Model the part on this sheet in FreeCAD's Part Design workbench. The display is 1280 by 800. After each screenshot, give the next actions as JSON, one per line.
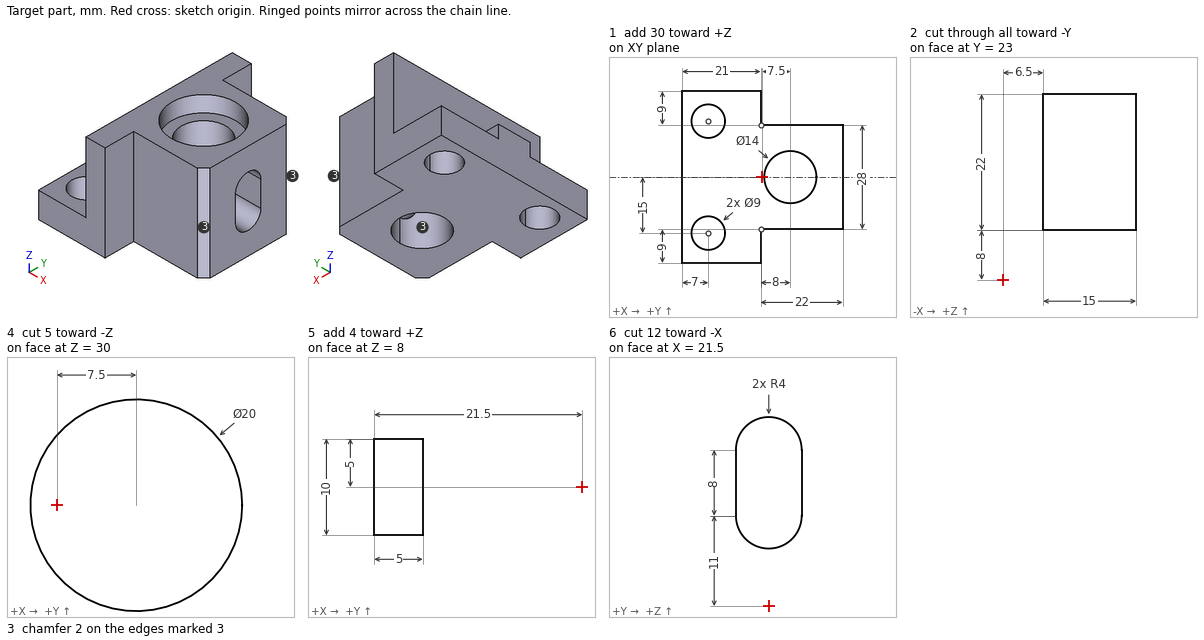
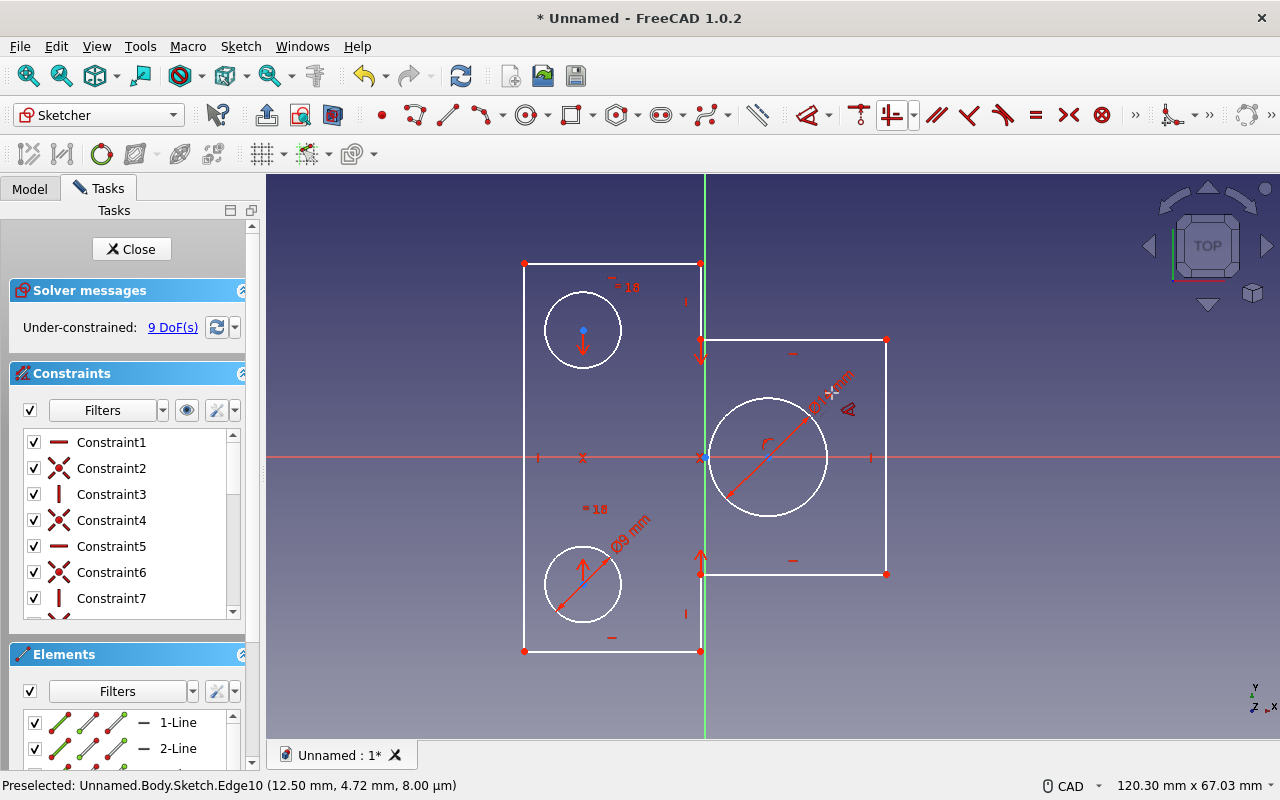
{"action": "scroll", "coordinate": [701, 317], "scroll_direction": "up", "scroll_amount": 6}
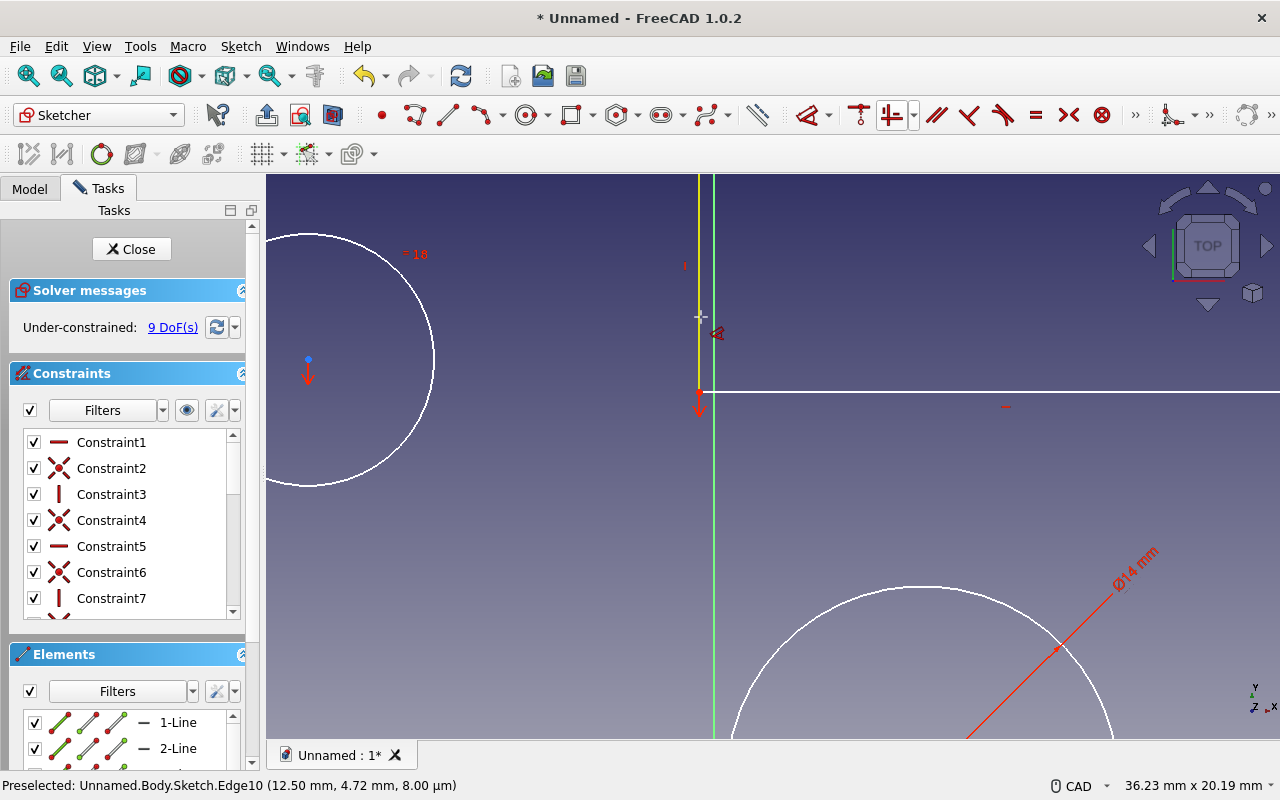
{"action": "left_click", "coordinate": [699, 316]}
{"action": "left_click", "coordinate": [665, 297]}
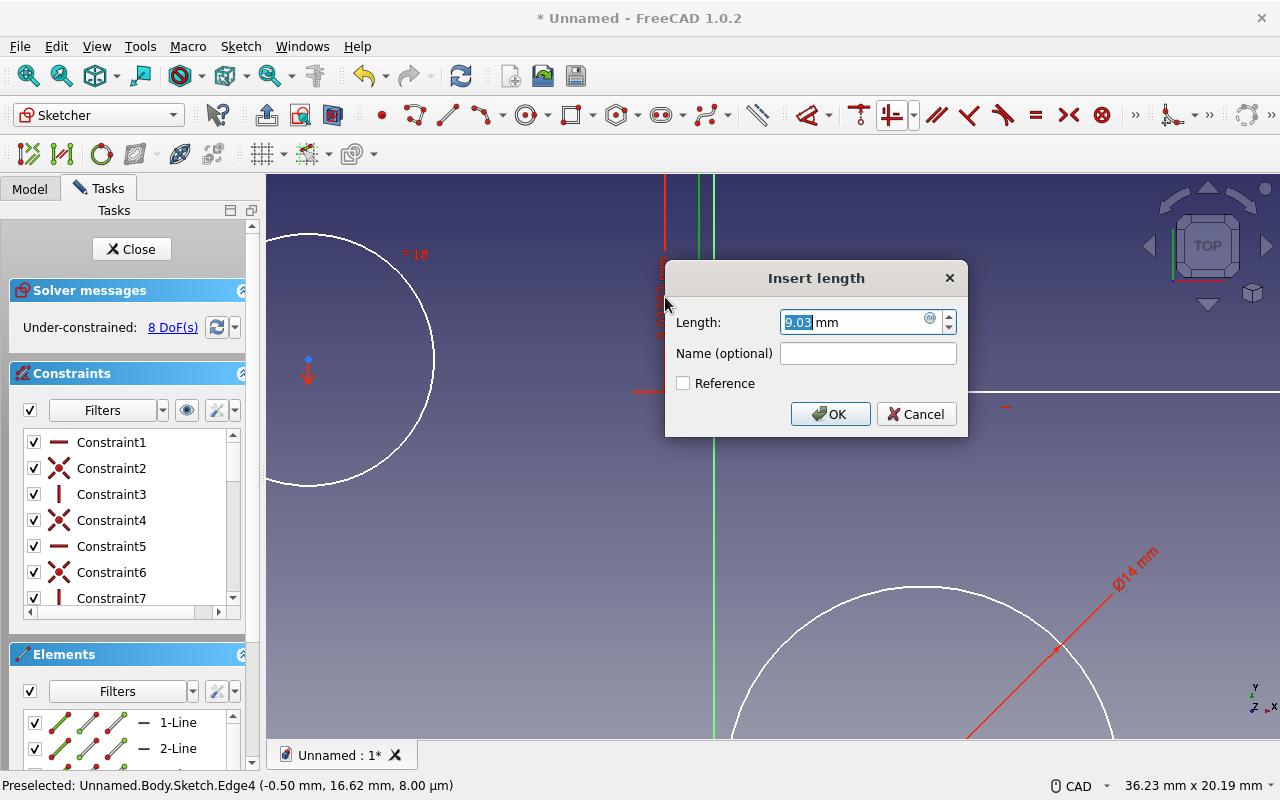
{"action": "type", "text": "9"}
{"action": "key", "text": "Return"}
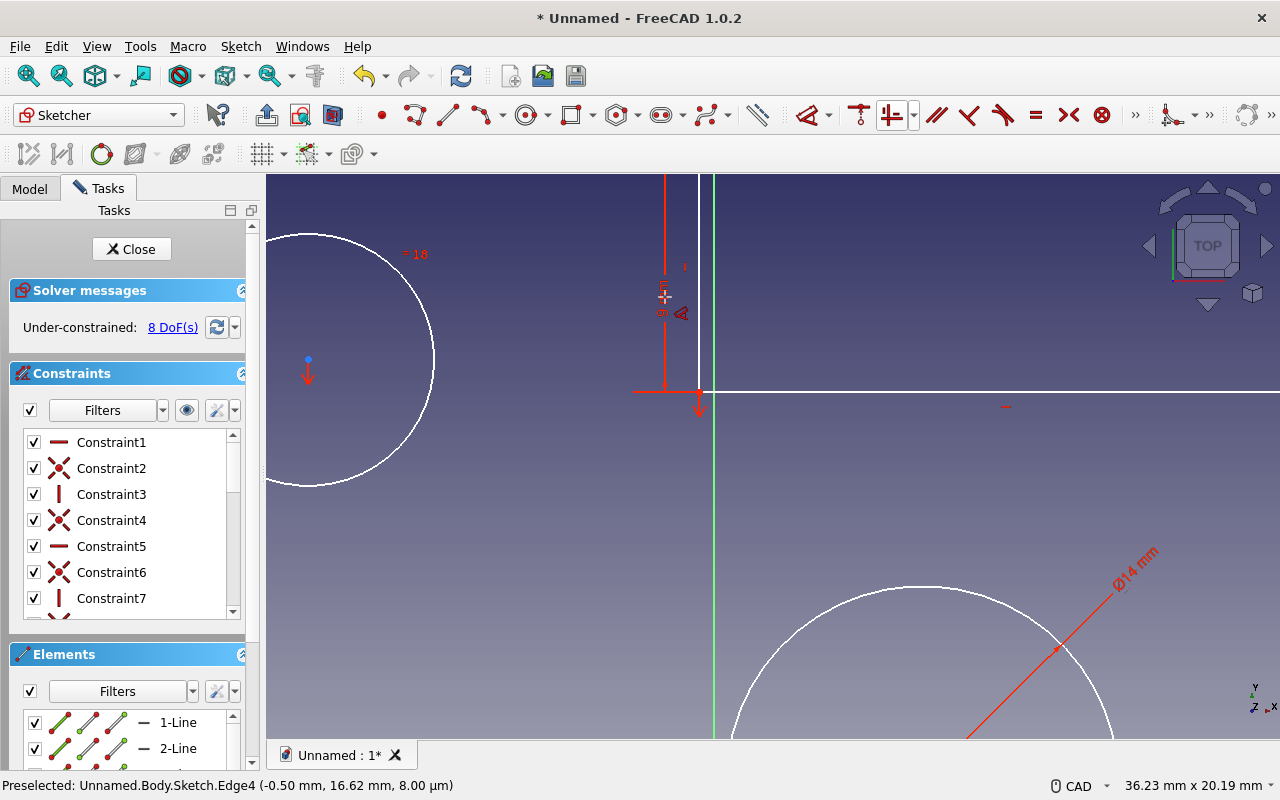
{"action": "scroll", "coordinate": [701, 316], "scroll_direction": "down", "scroll_amount": 6}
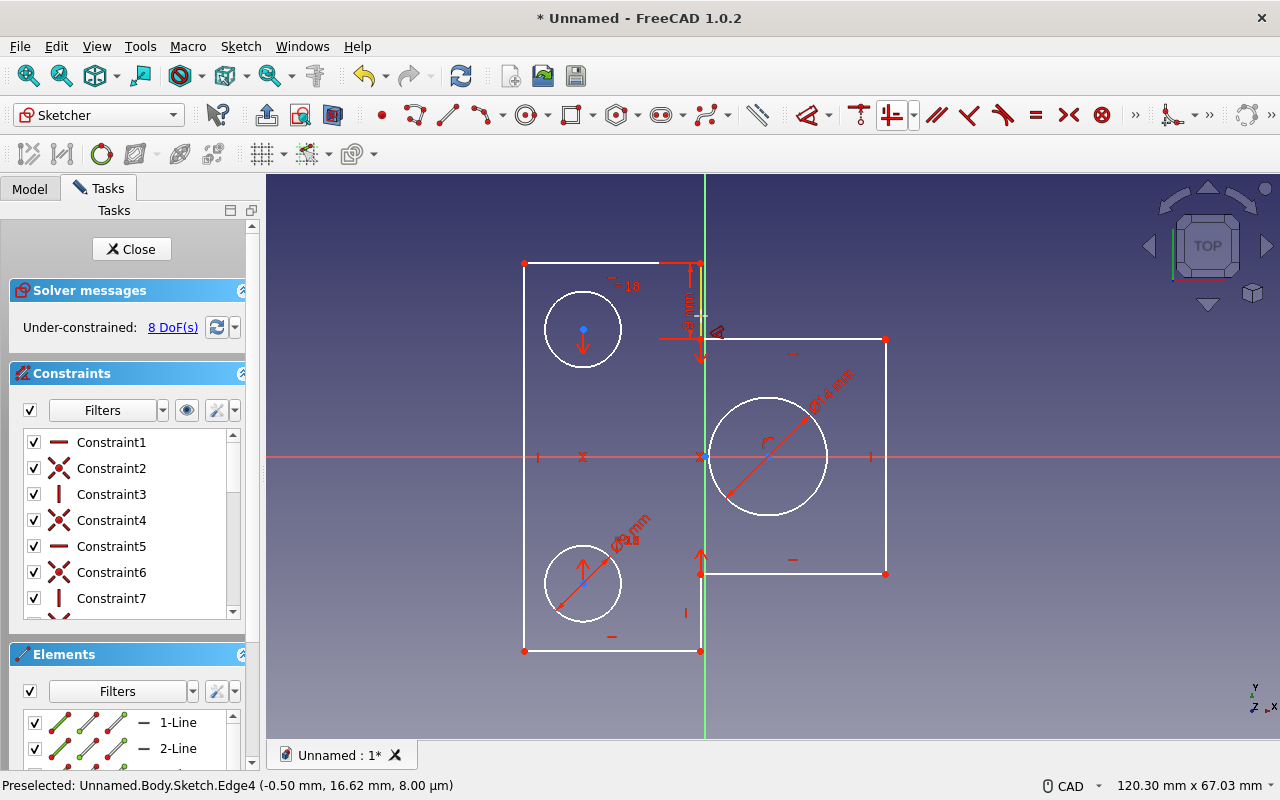
{"action": "scroll", "coordinate": [701, 628], "scroll_direction": "up", "scroll_amount": 6}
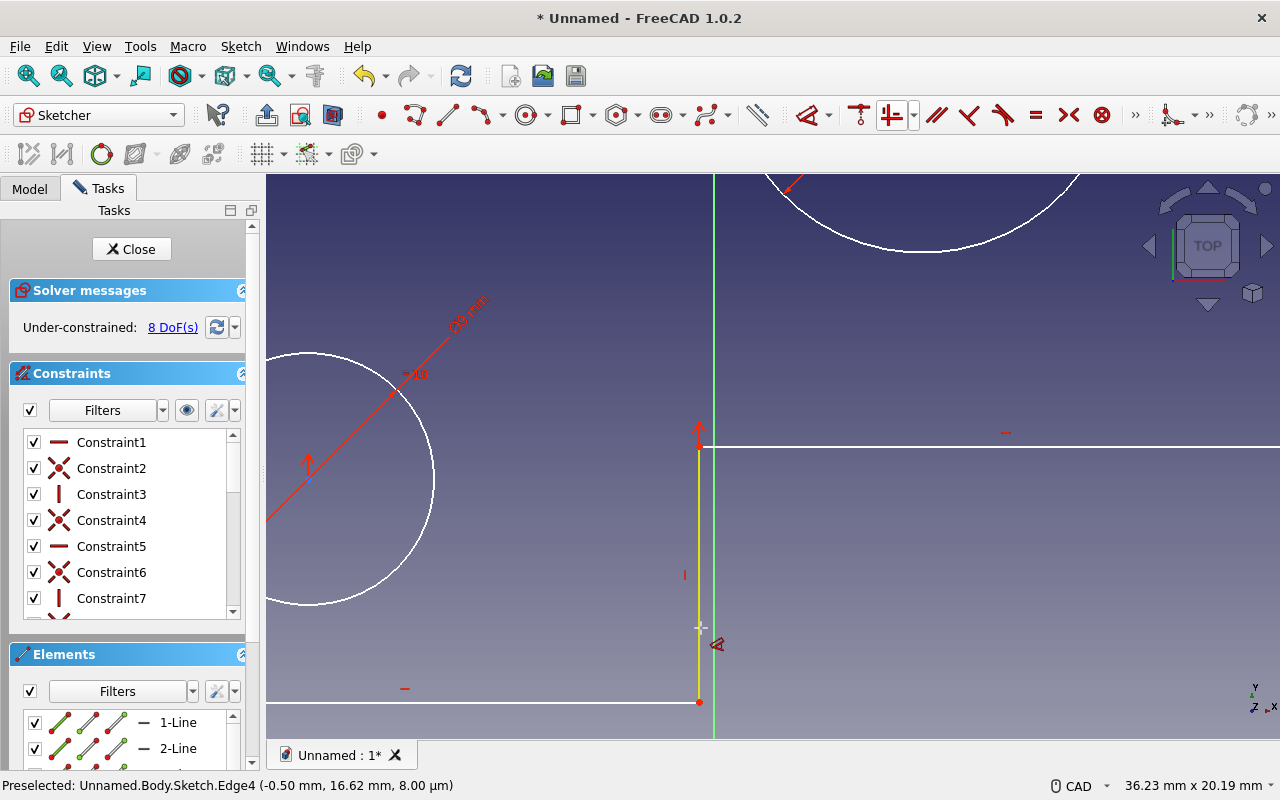
{"action": "left_click", "coordinate": [699, 626]}
{"action": "left_click", "coordinate": [665, 575]}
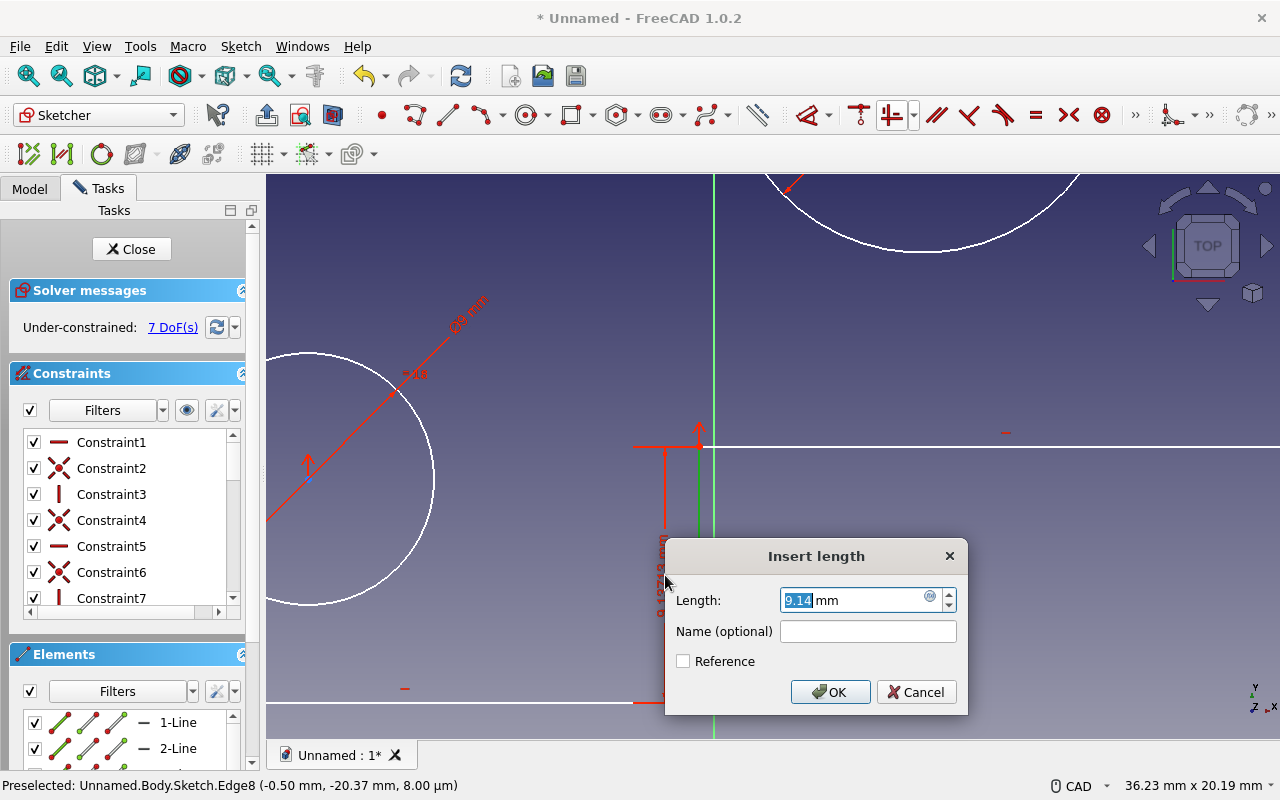
{"action": "type", "text": "9"}
{"action": "key", "text": "Return"}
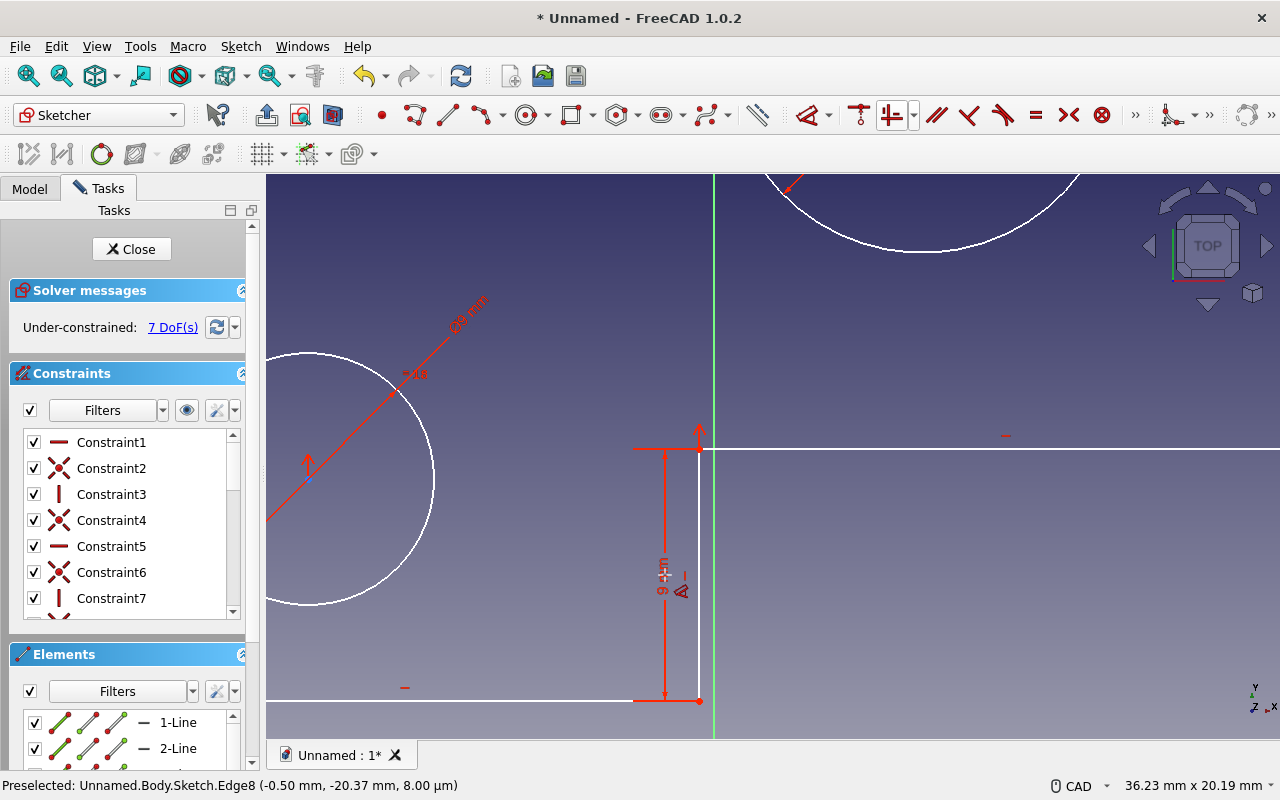
{"action": "left_click", "coordinate": [884, 449]}
{"action": "left_click", "coordinate": [907, 483]}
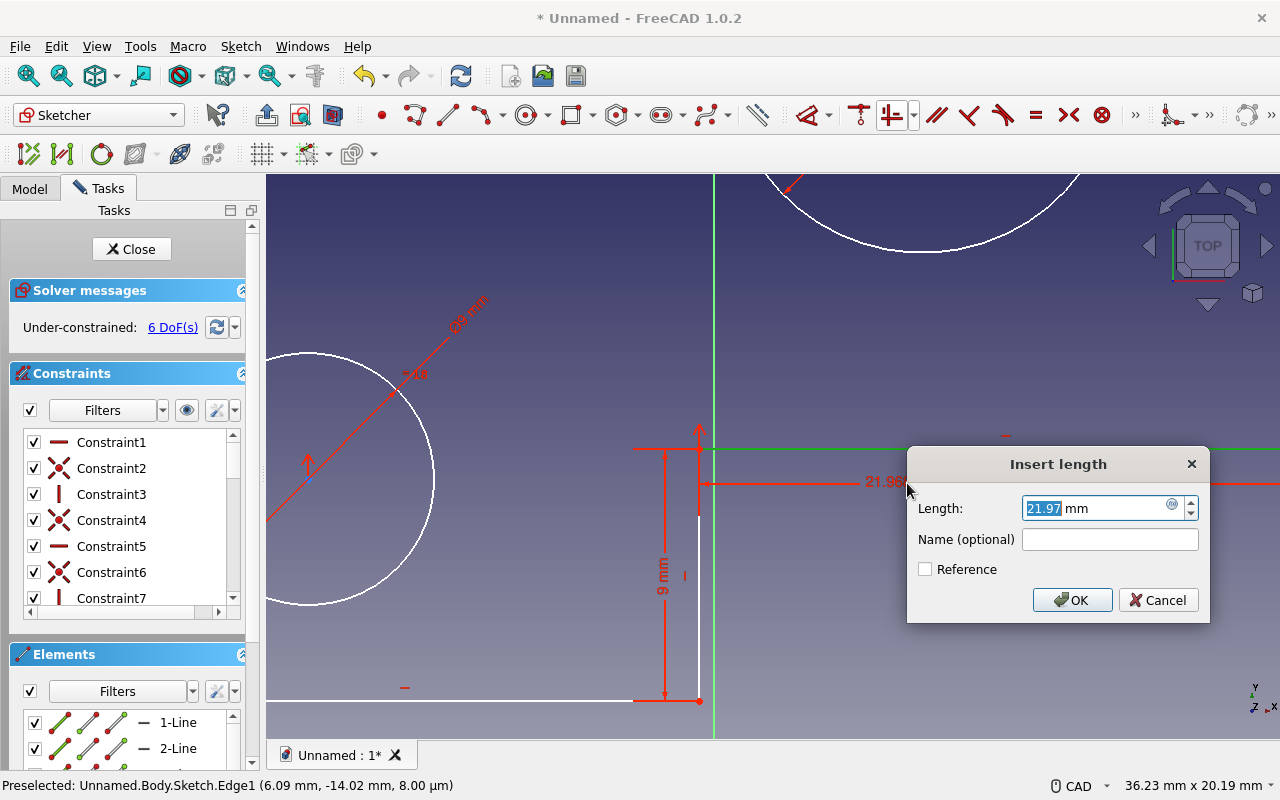
{"action": "type", "text": "22"}
{"action": "key", "text": "Return"}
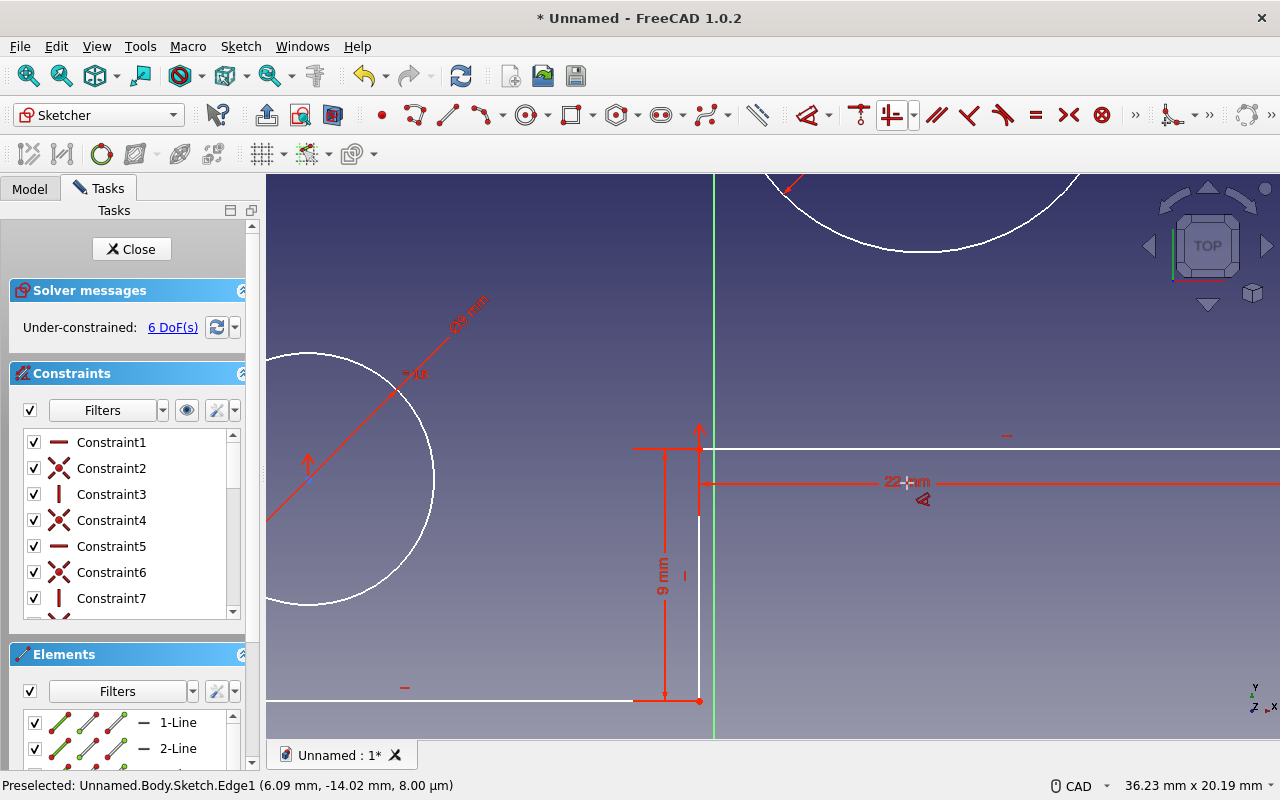
{"action": "scroll", "coordinate": [701, 629], "scroll_direction": "down", "scroll_amount": 6}